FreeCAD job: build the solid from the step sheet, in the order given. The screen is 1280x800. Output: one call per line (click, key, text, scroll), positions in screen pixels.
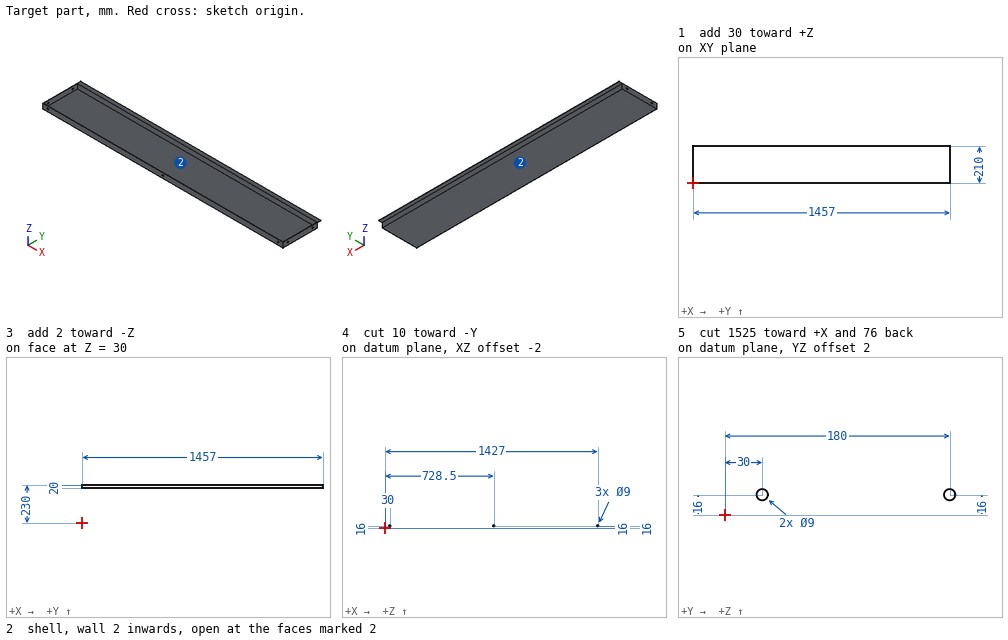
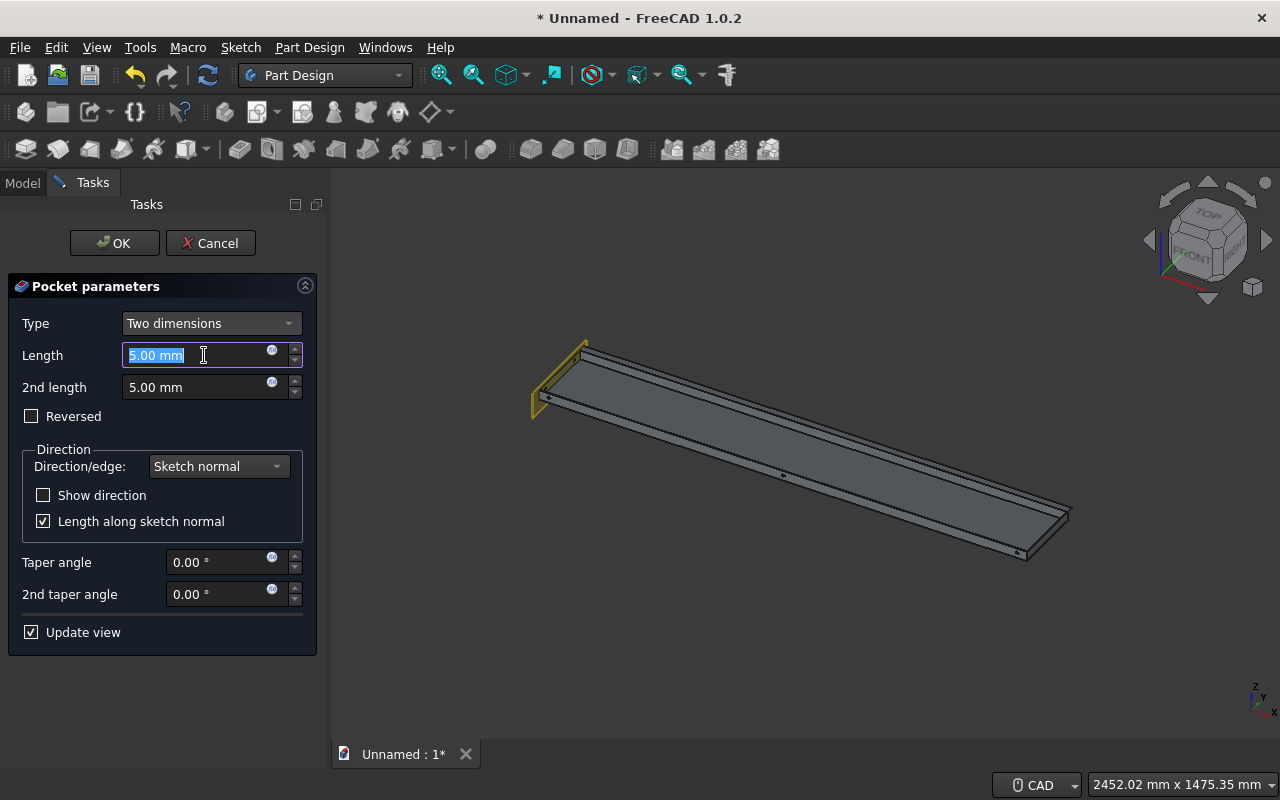
text(1525)
key(Tab)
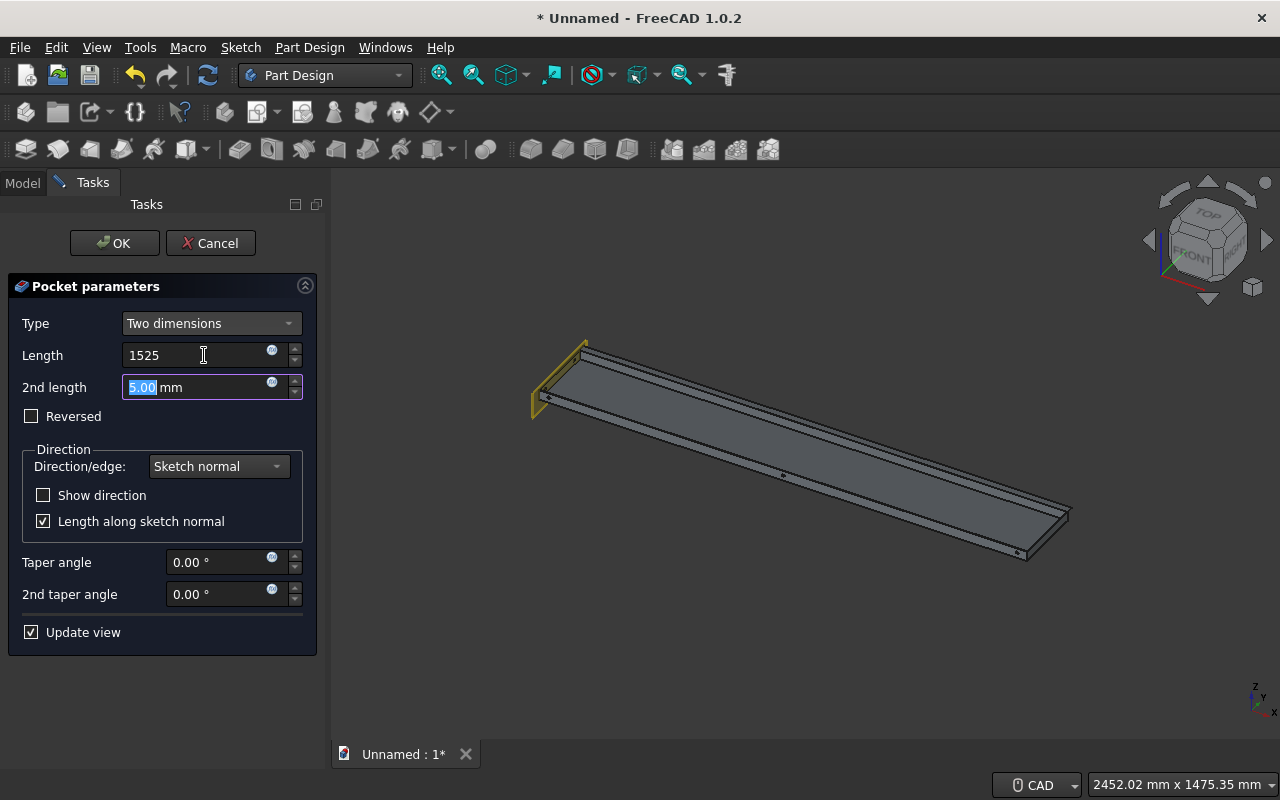
text(76)
key(Tab)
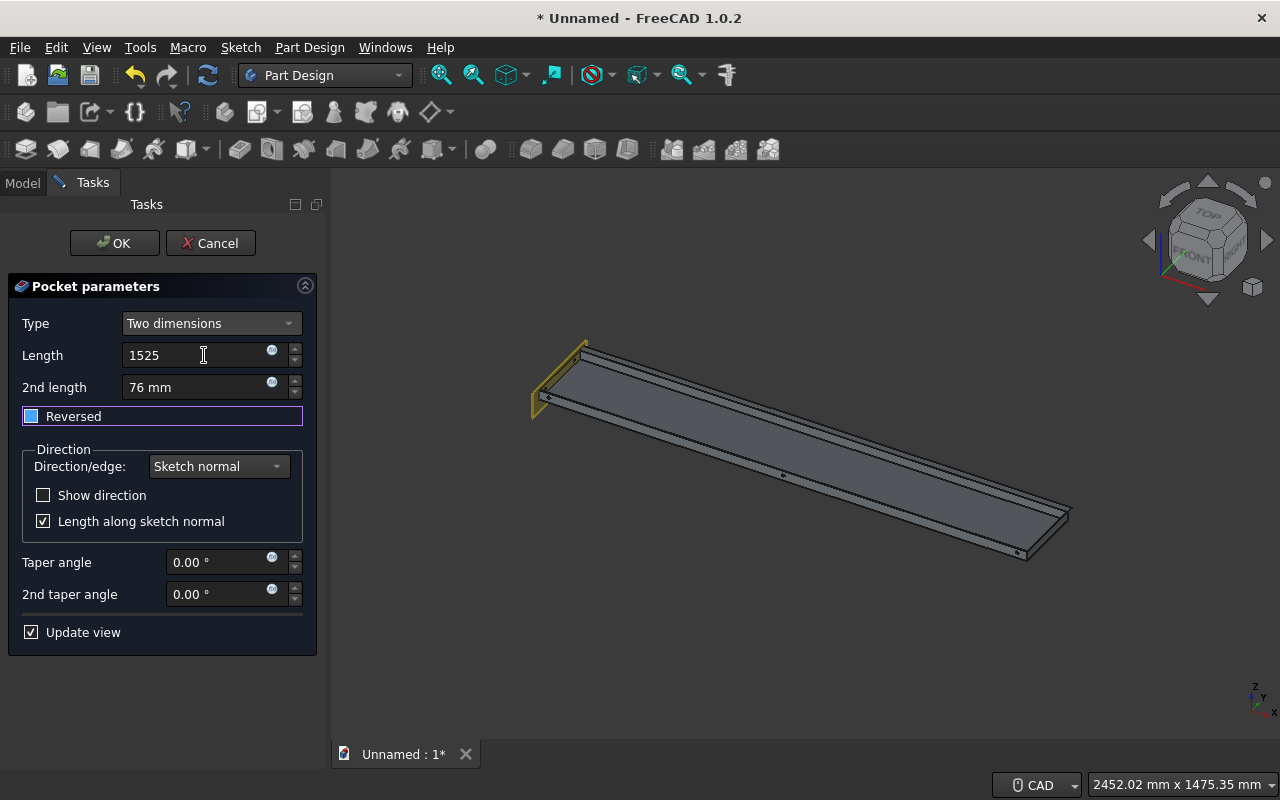
click(30, 416)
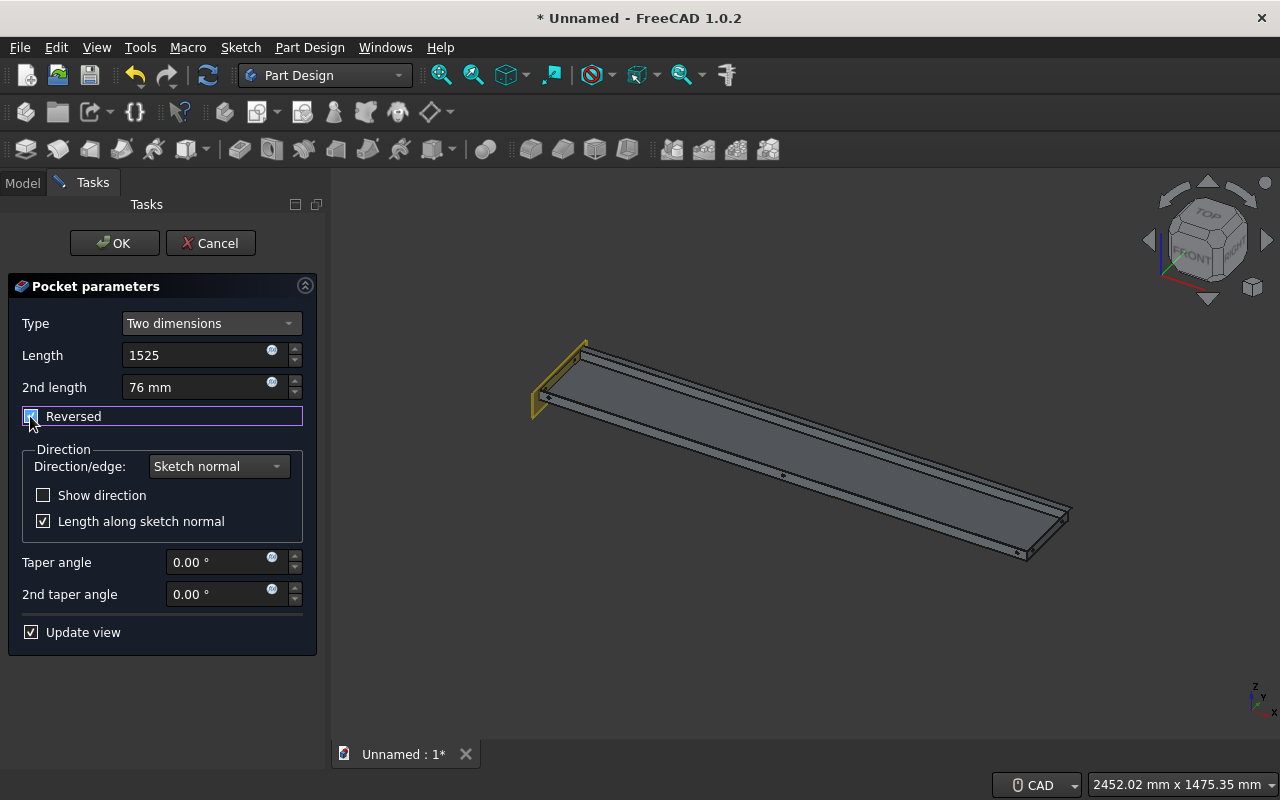
click(115, 243)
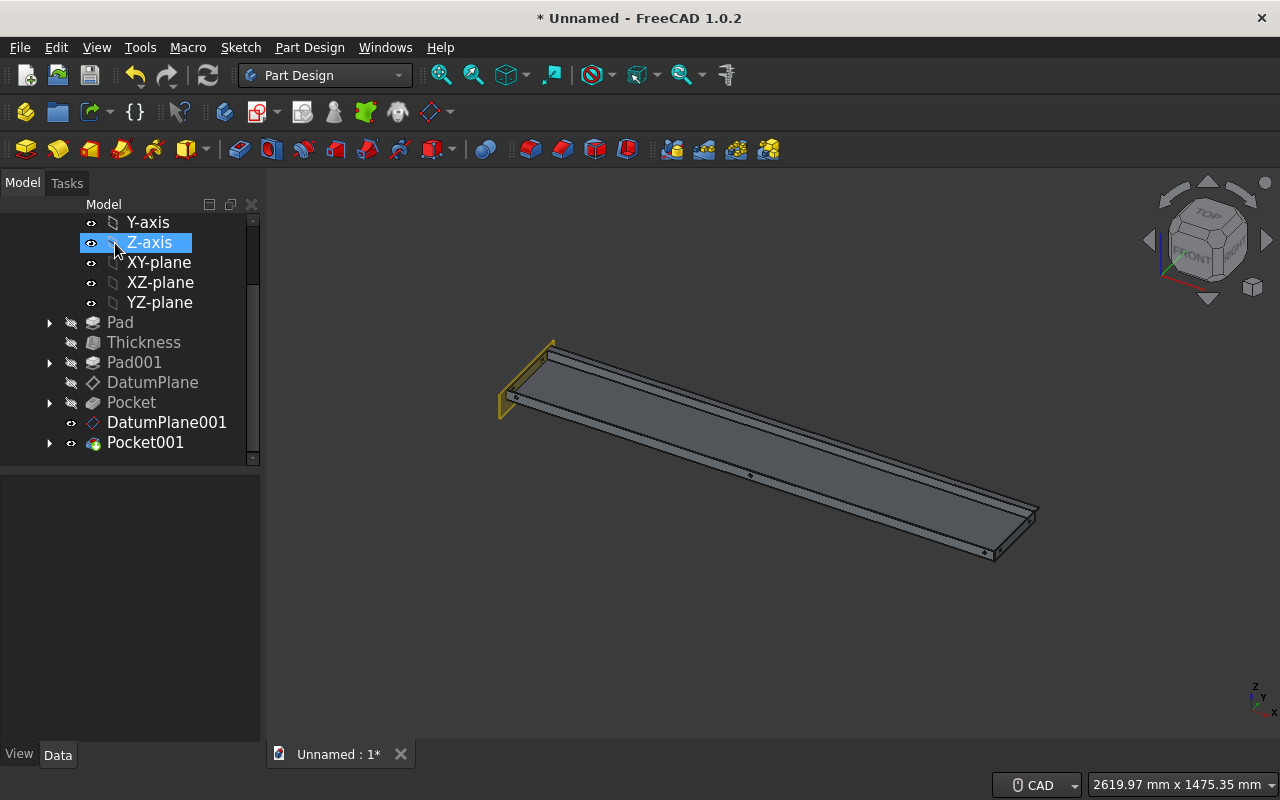
click(116, 423)
key(space)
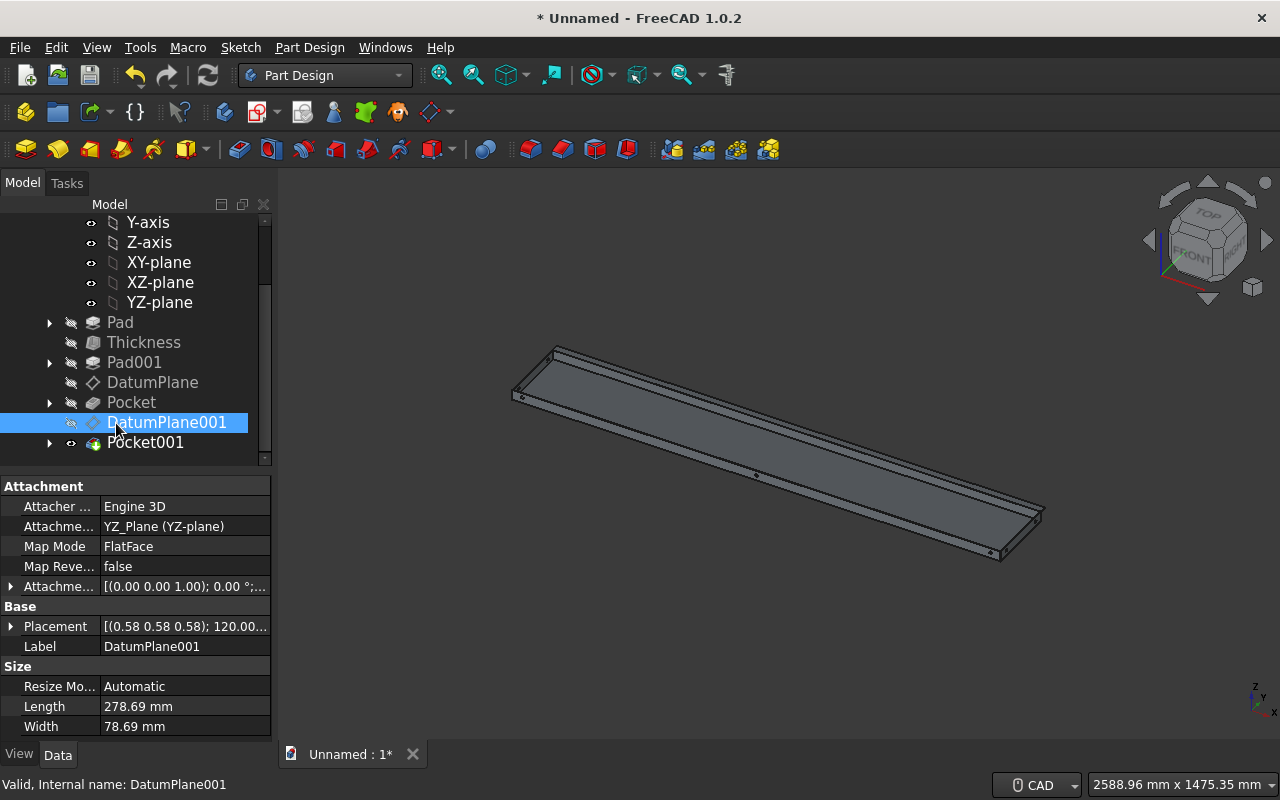
key(0)